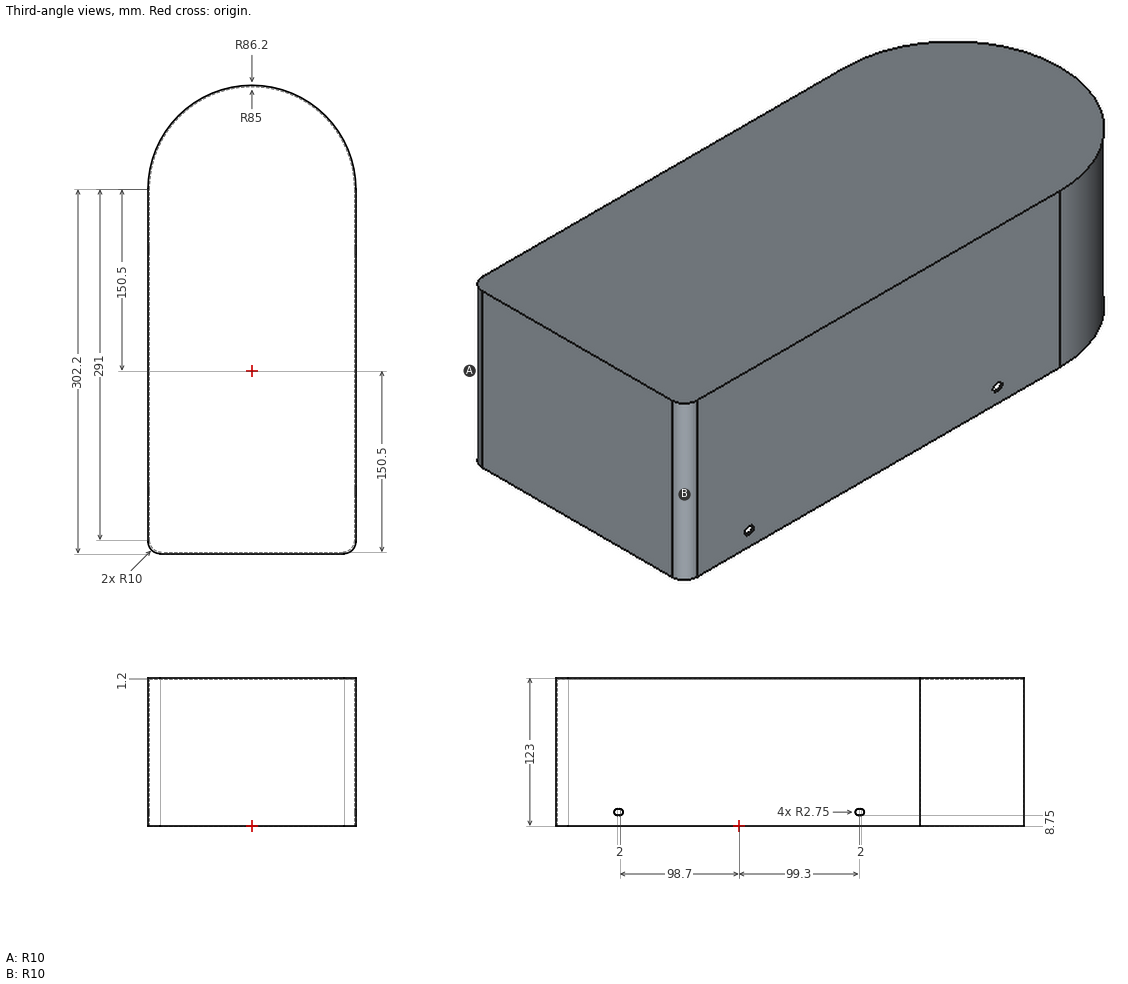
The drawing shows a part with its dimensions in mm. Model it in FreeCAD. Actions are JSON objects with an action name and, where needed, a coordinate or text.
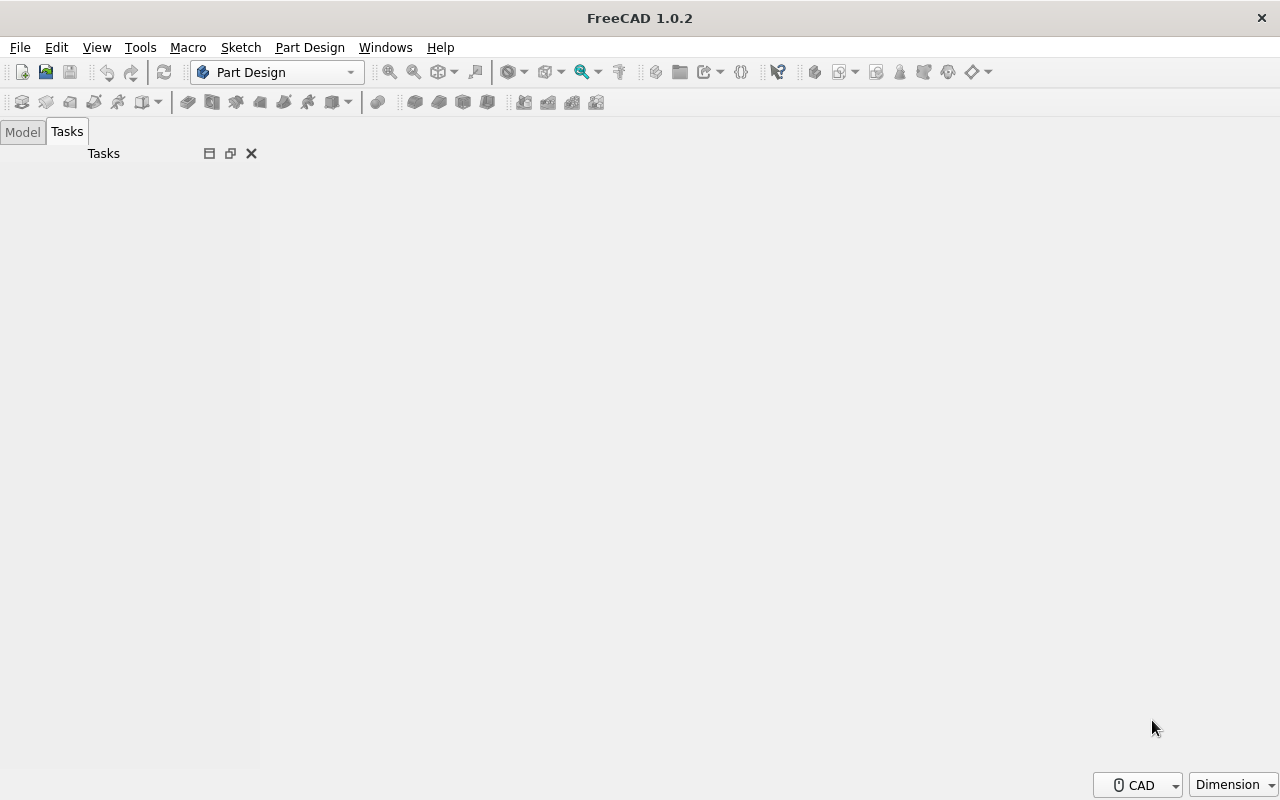
{"action": "key", "text": "ctrl+n"}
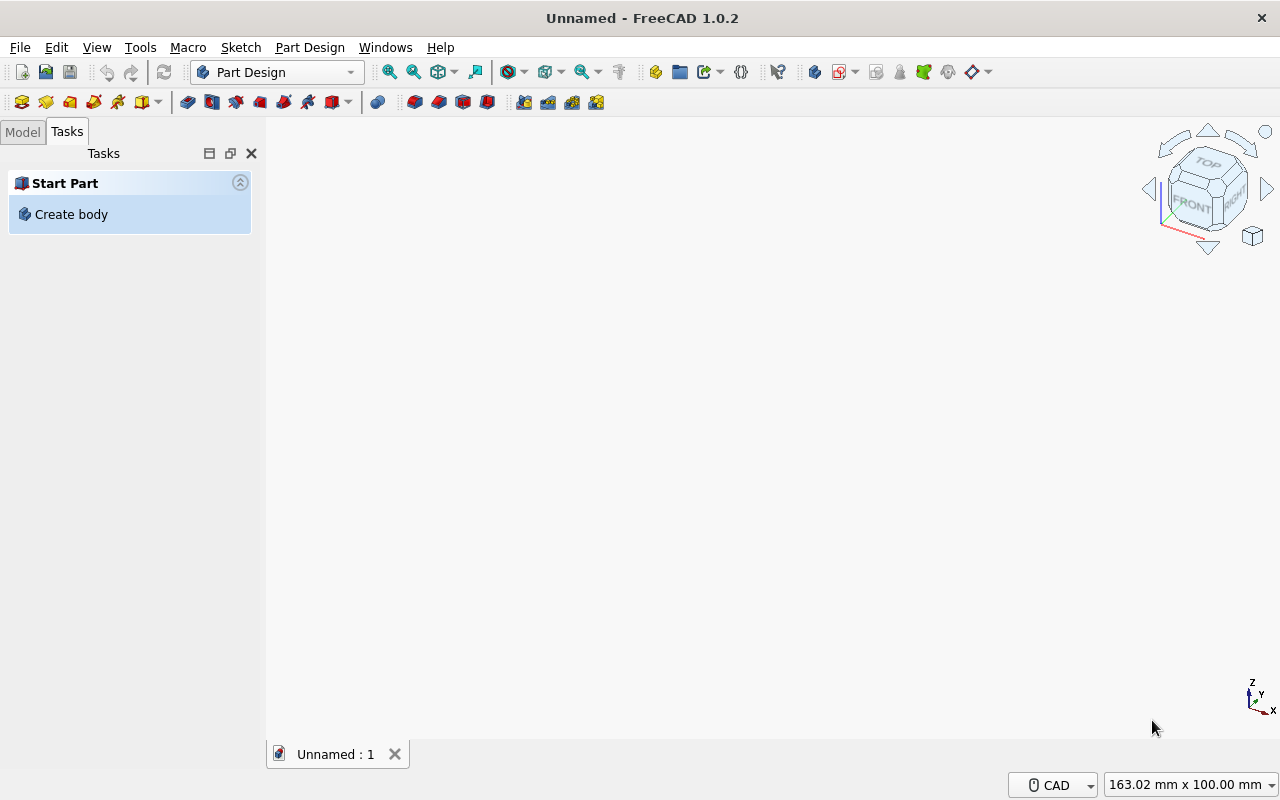
{"action": "left_click", "coordinate": [840, 72]}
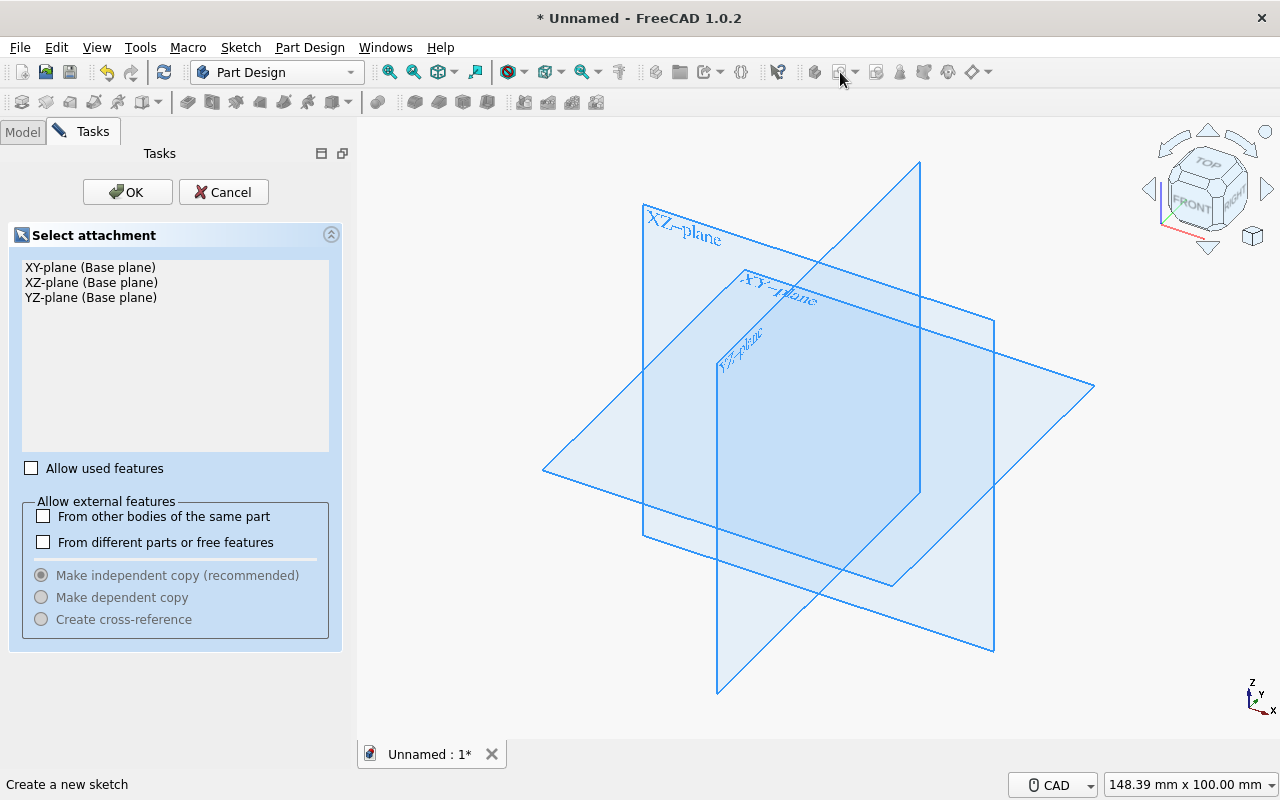
{"action": "left_click", "coordinate": [82, 268]}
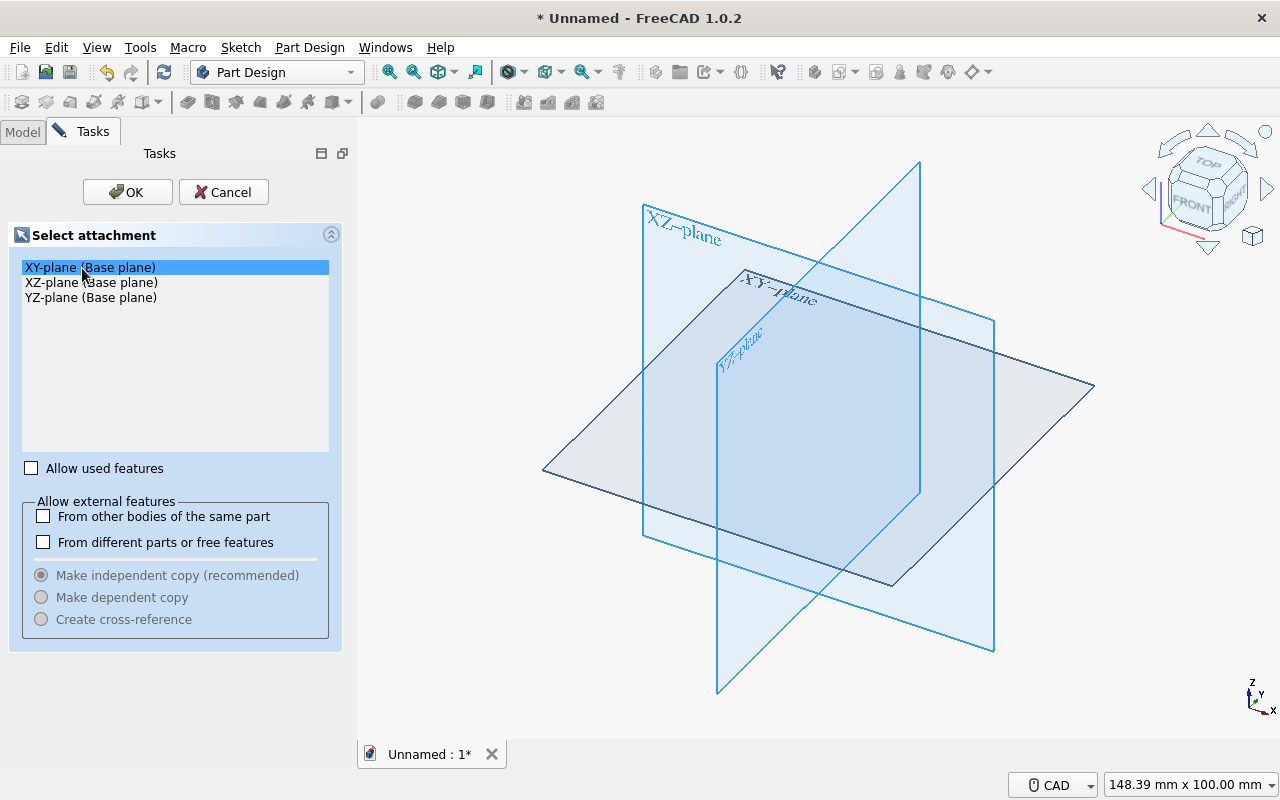
{"action": "left_click", "coordinate": [128, 192]}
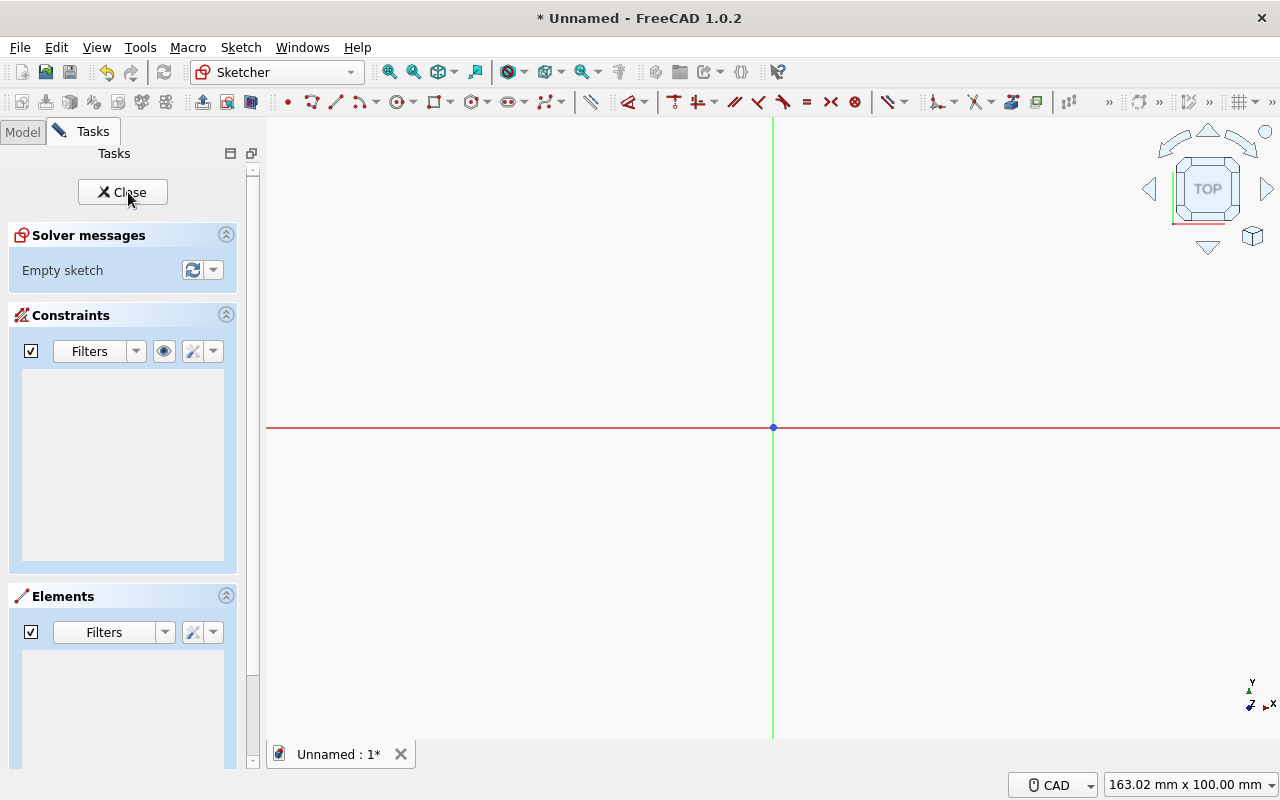
{"action": "scroll", "coordinate": [691, 480], "scroll_direction": "down", "scroll_amount": 9}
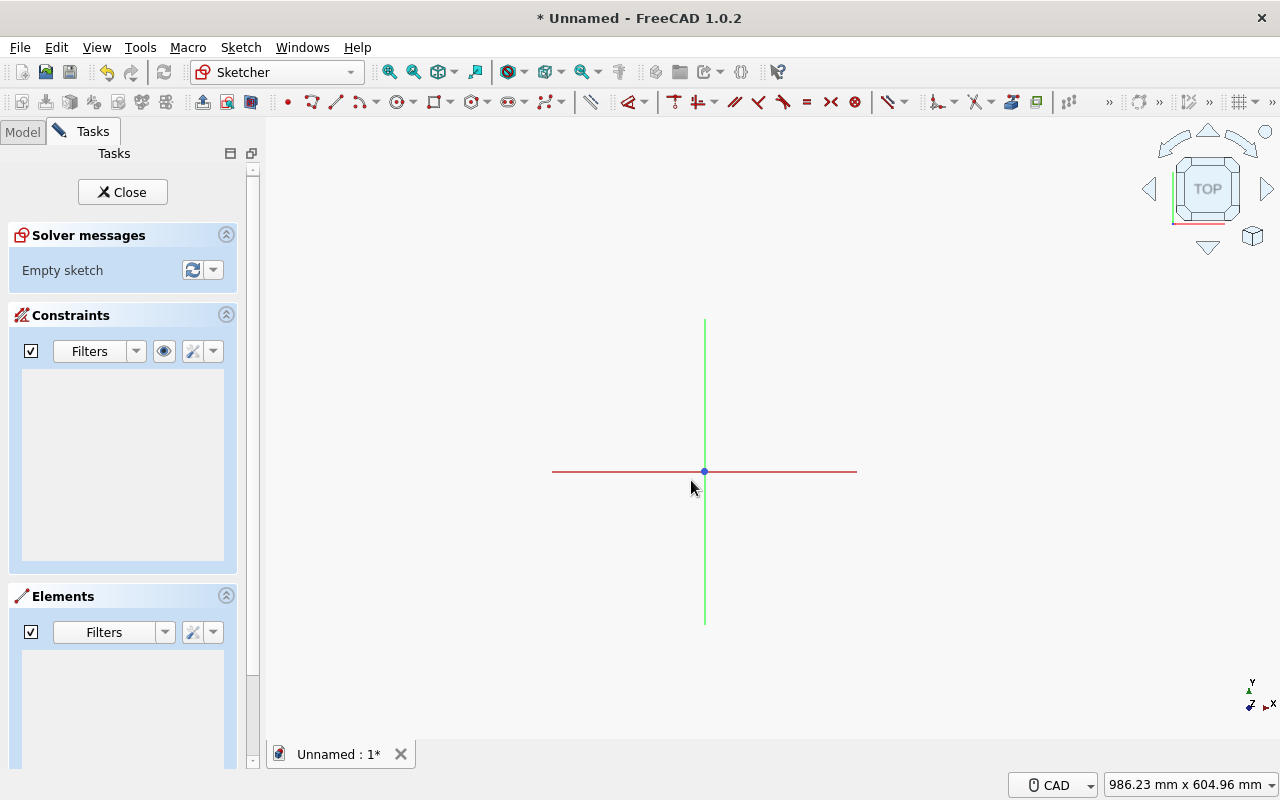
{"action": "left_click", "coordinate": [312, 102]}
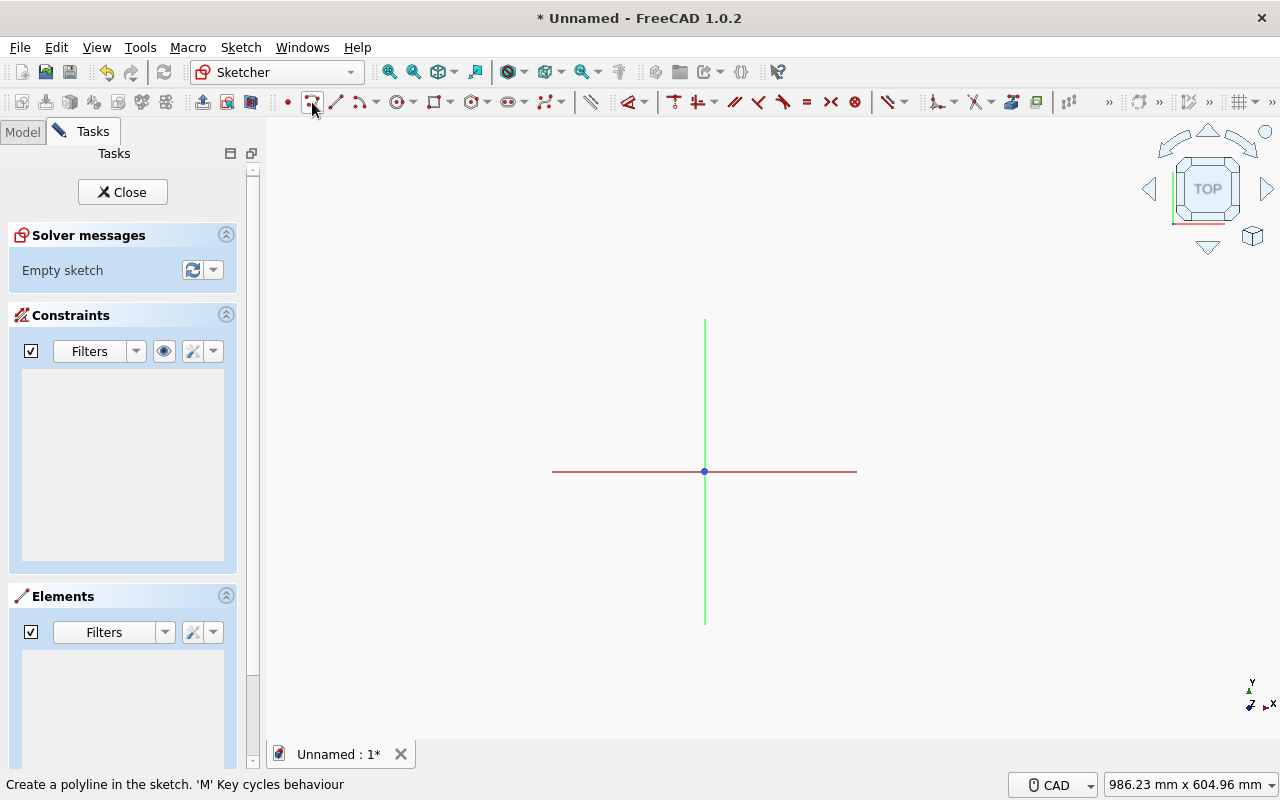
{"action": "left_click", "coordinate": [616, 317]}
{"action": "left_click", "coordinate": [616, 628]}
{"action": "left_click", "coordinate": [794, 628]}
{"action": "left_click", "coordinate": [794, 317]}
{"action": "right_click", "coordinate": [794, 317]}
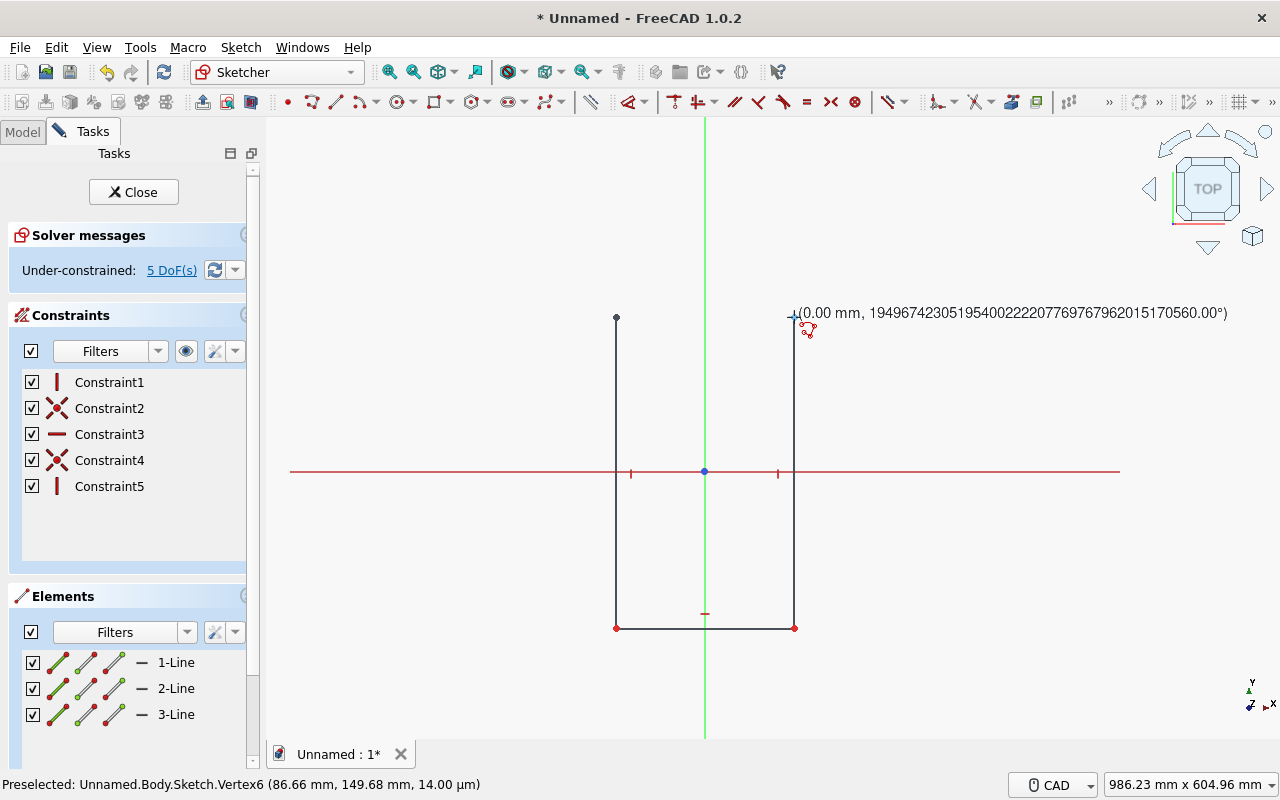
{"action": "left_click", "coordinate": [378, 102]}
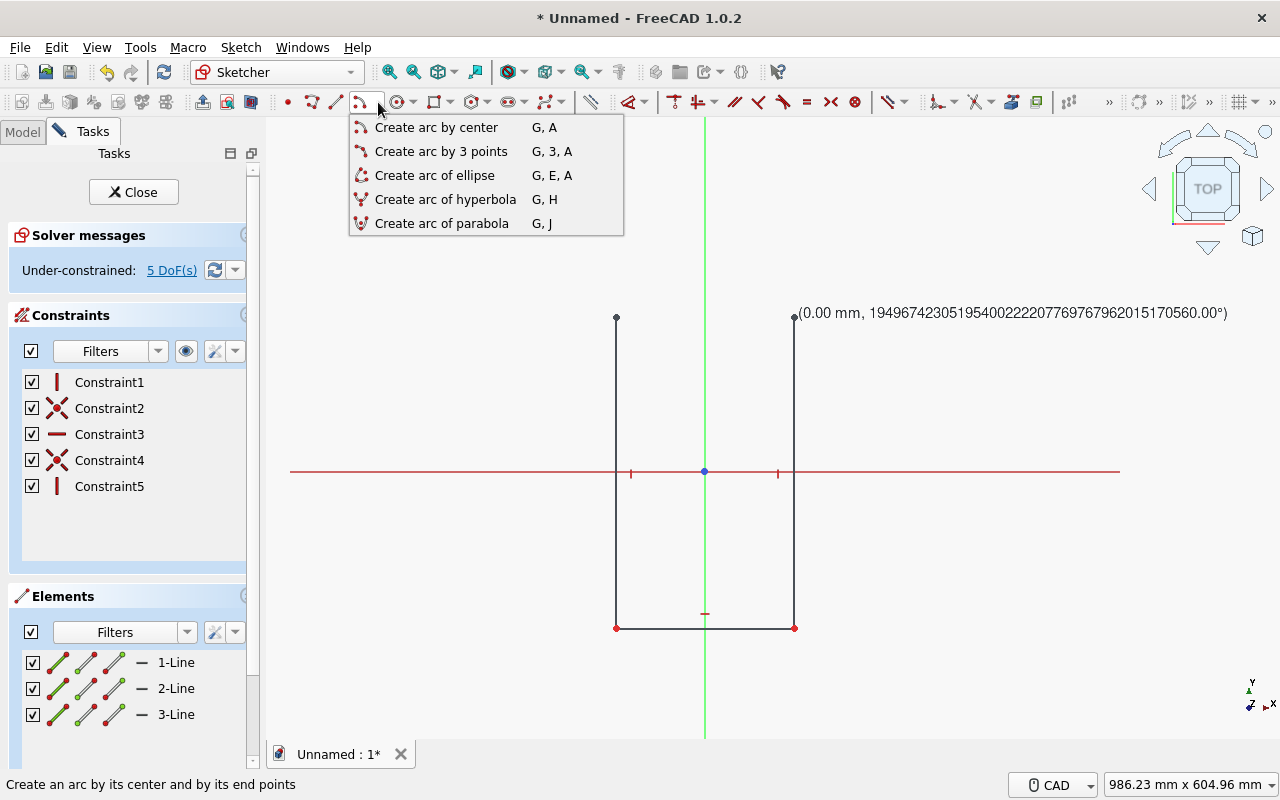
{"action": "left_click", "coordinate": [486, 151]}